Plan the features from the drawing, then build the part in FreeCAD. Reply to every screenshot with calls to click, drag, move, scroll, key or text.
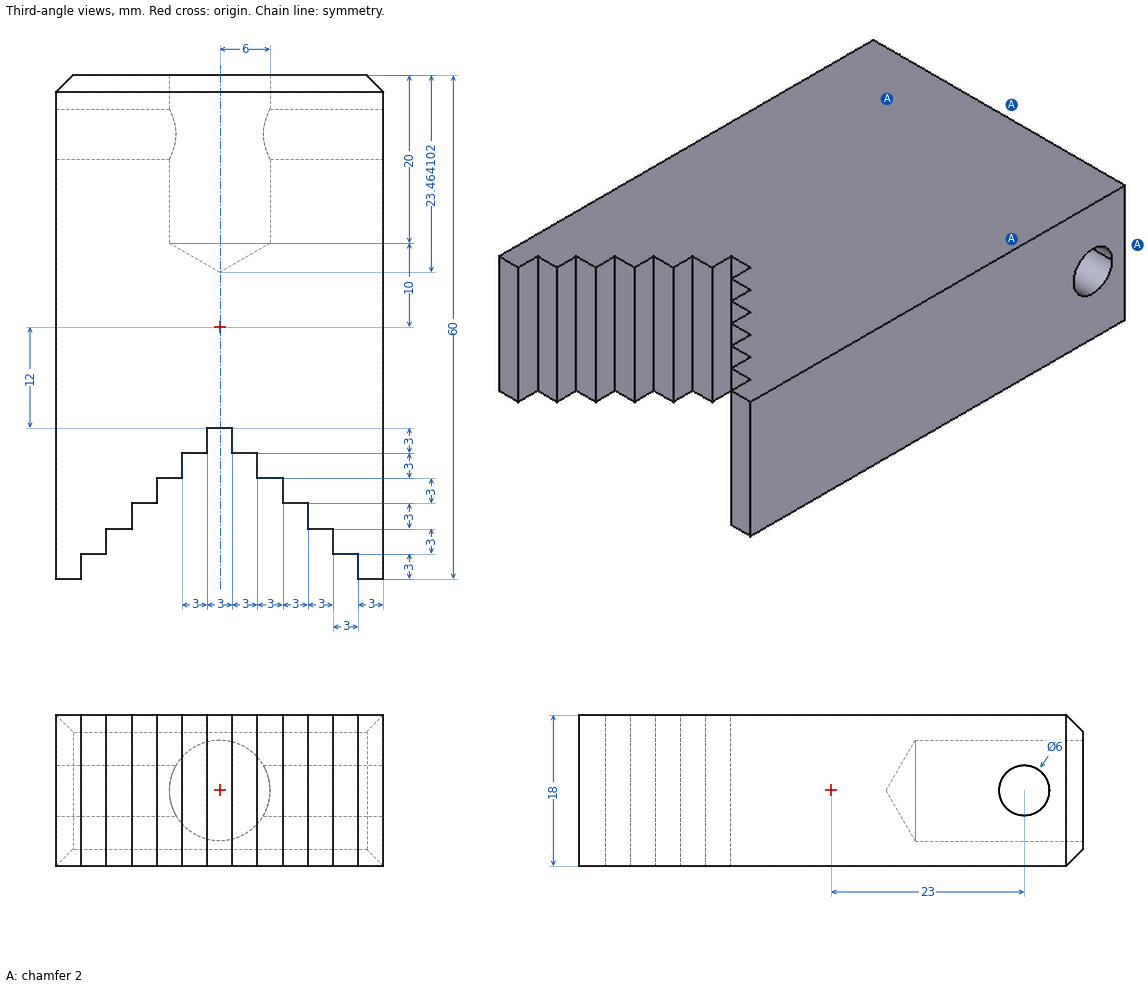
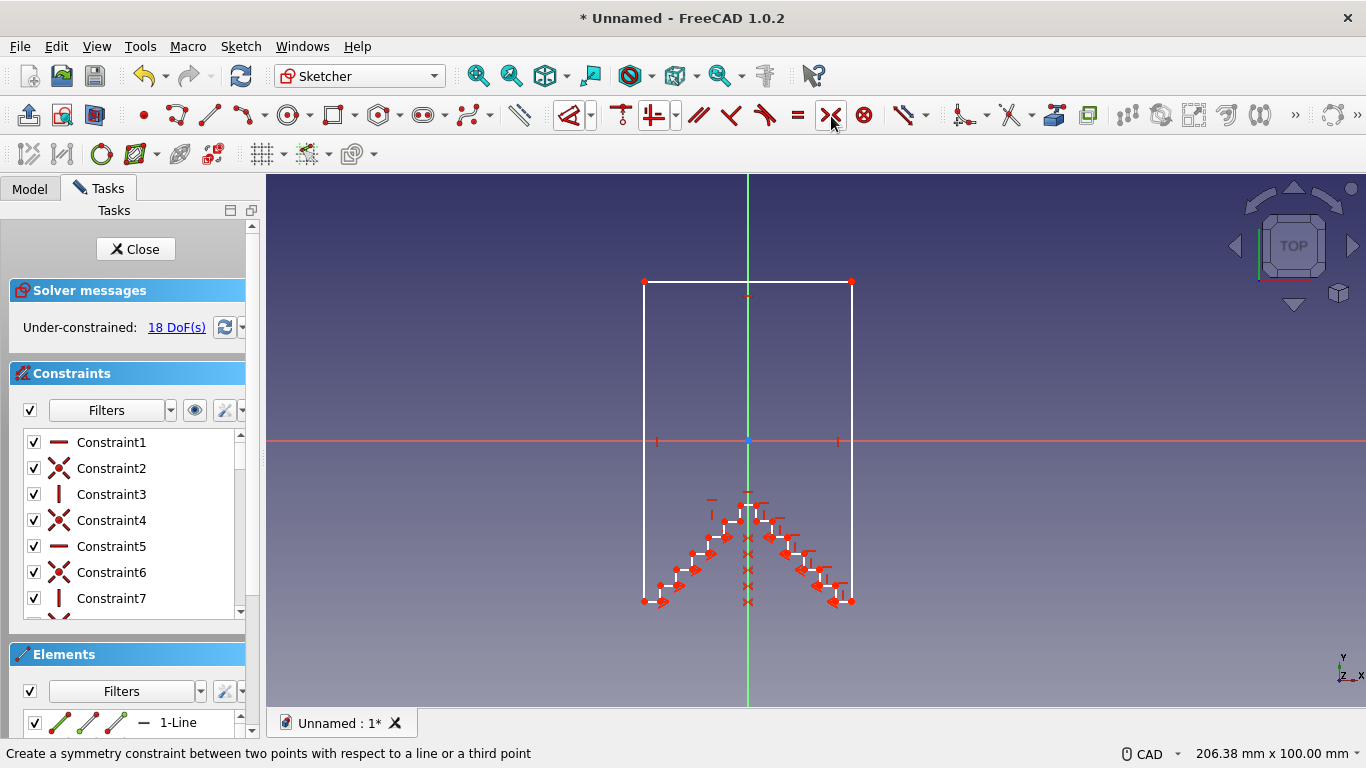
click(772, 521)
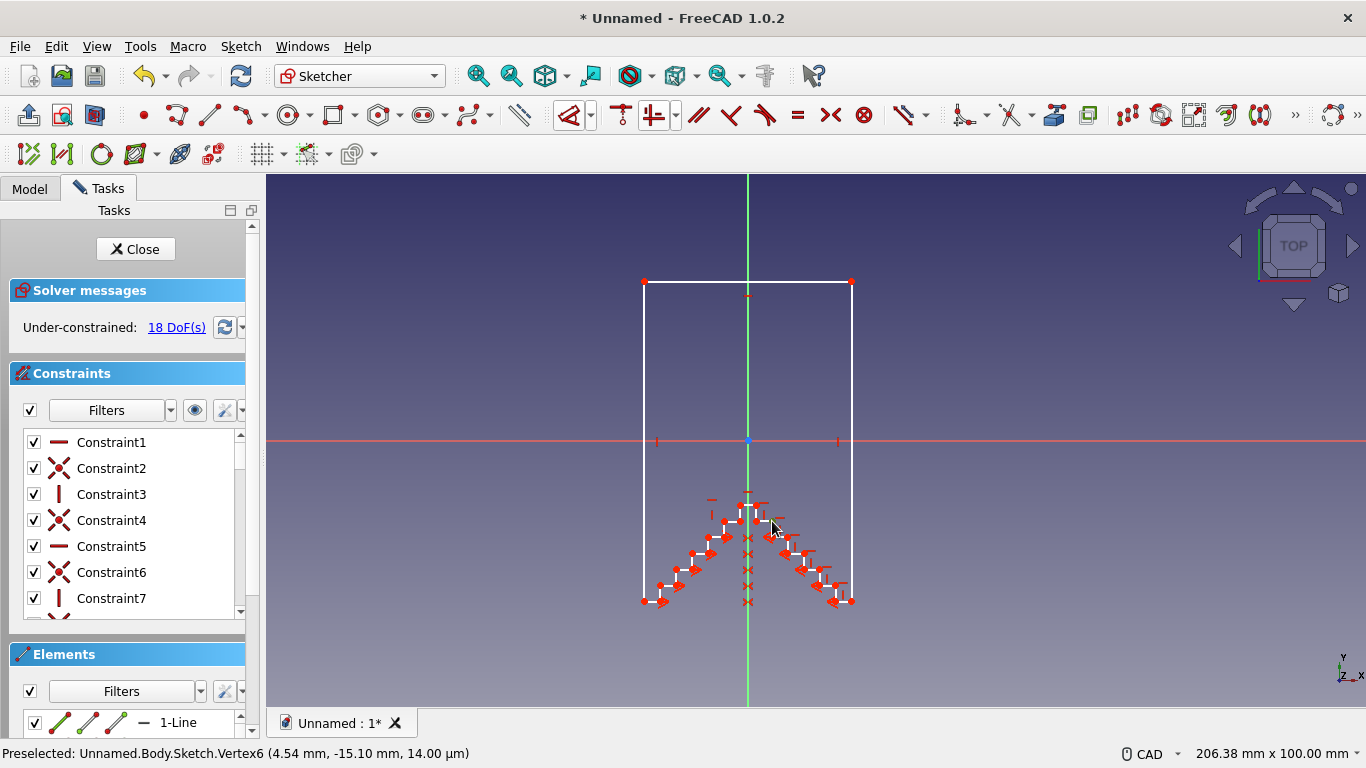
click(724, 522)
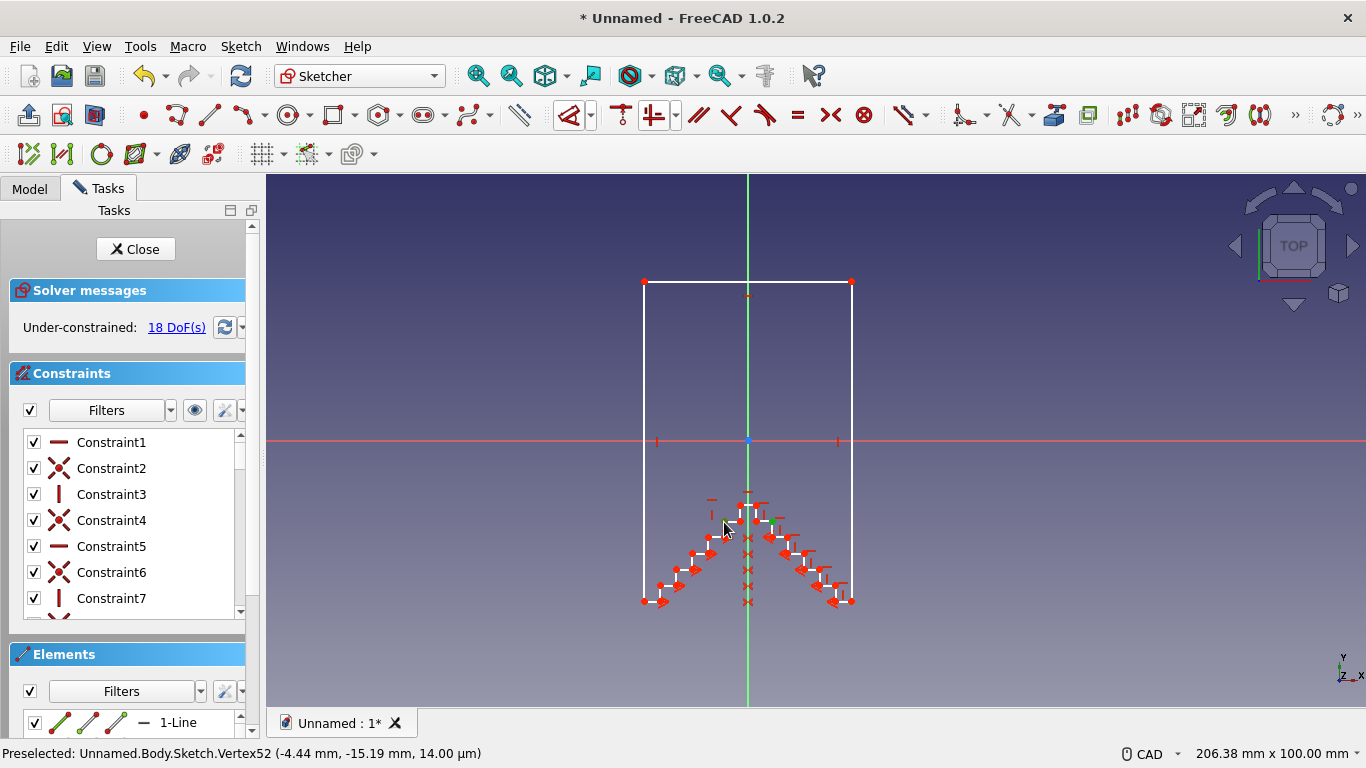
click(748, 645)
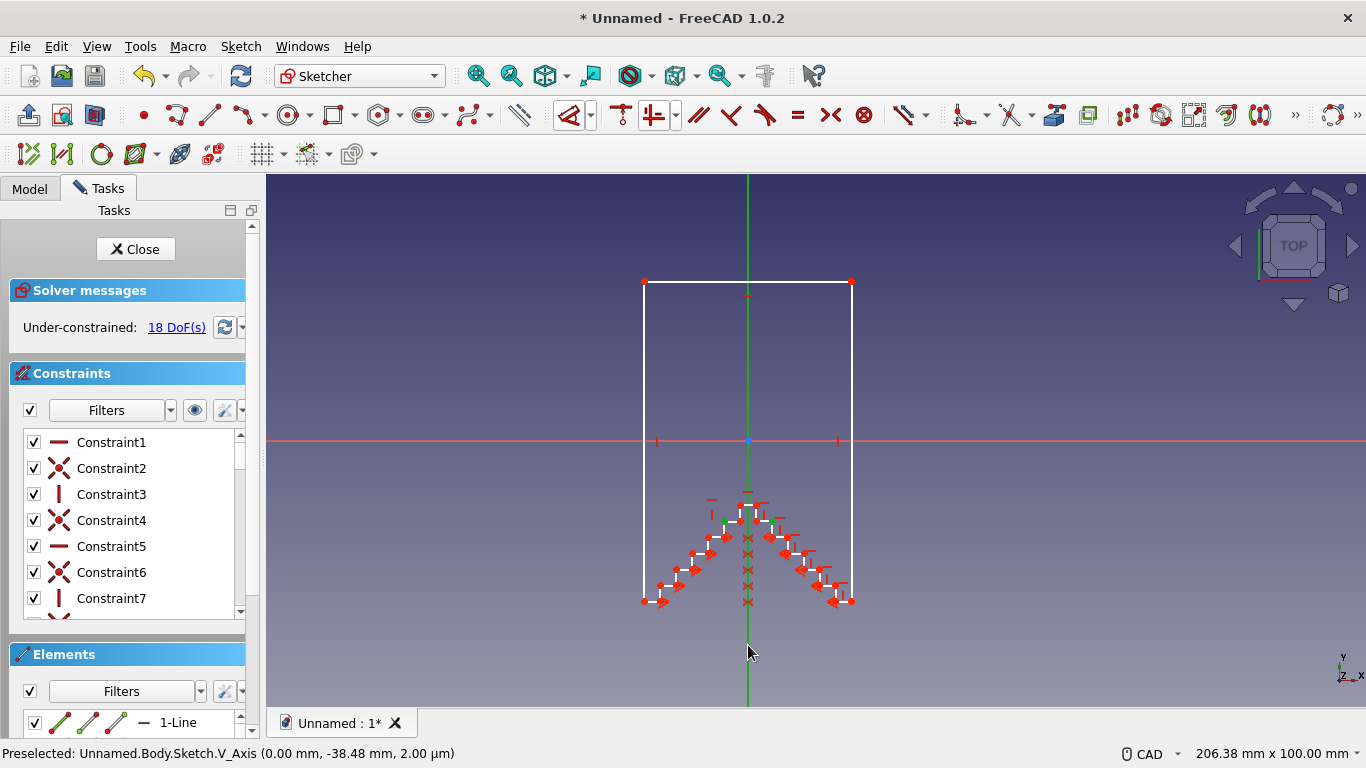
click(831, 116)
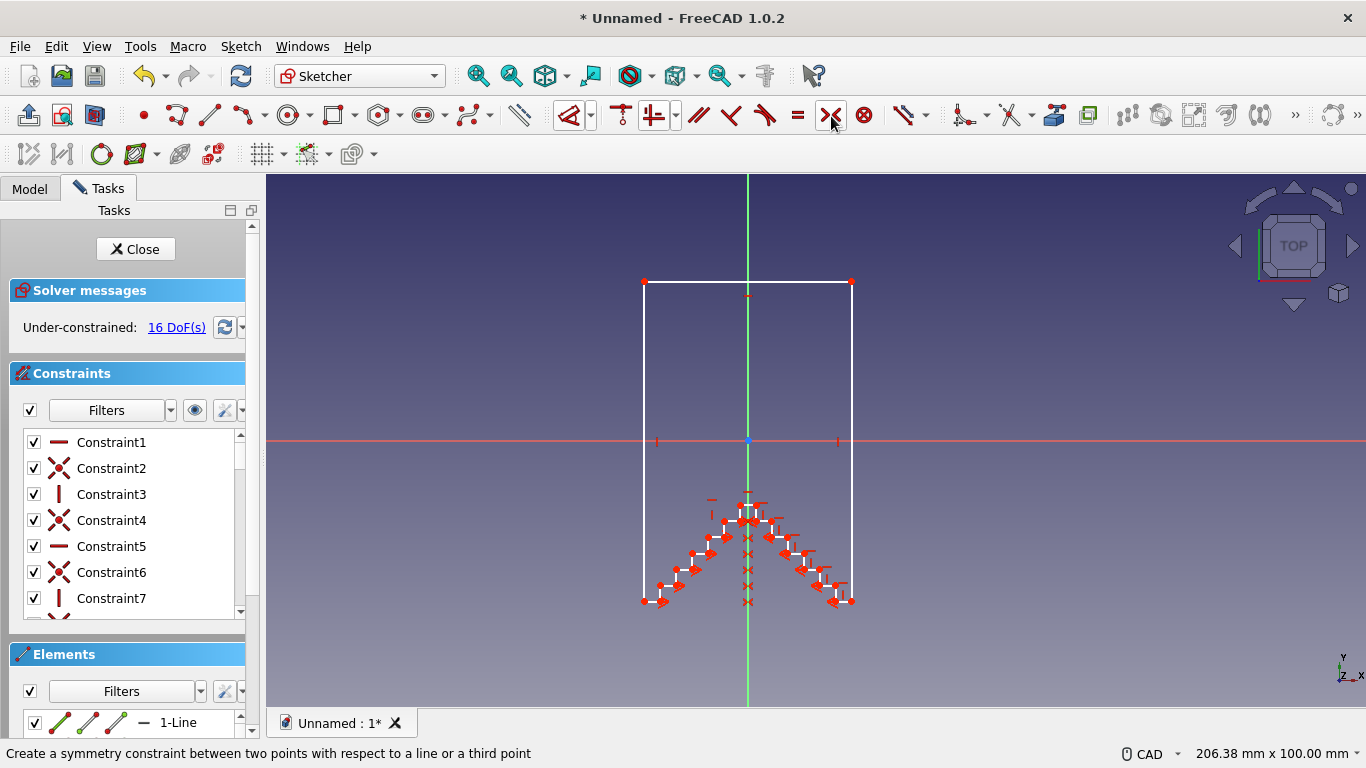
click(568, 116)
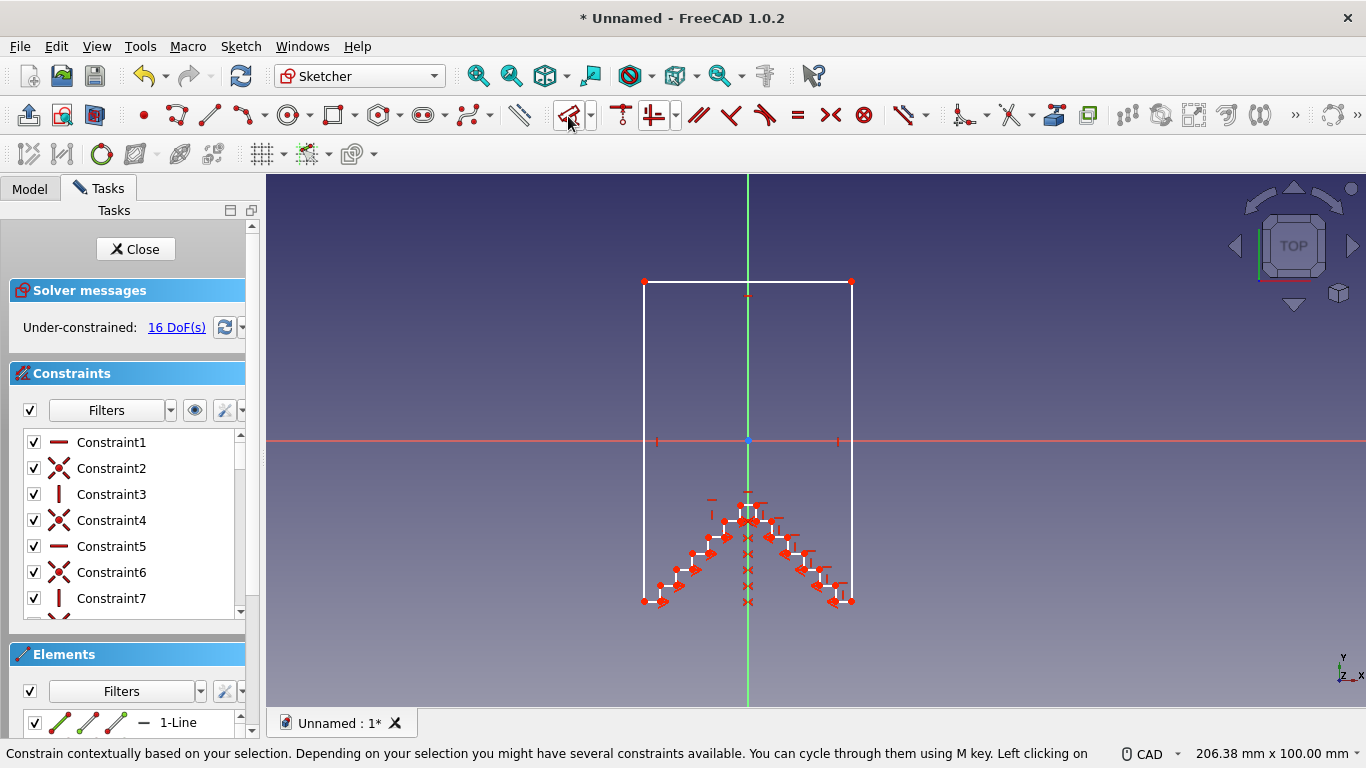
scroll(748, 505, up, 5)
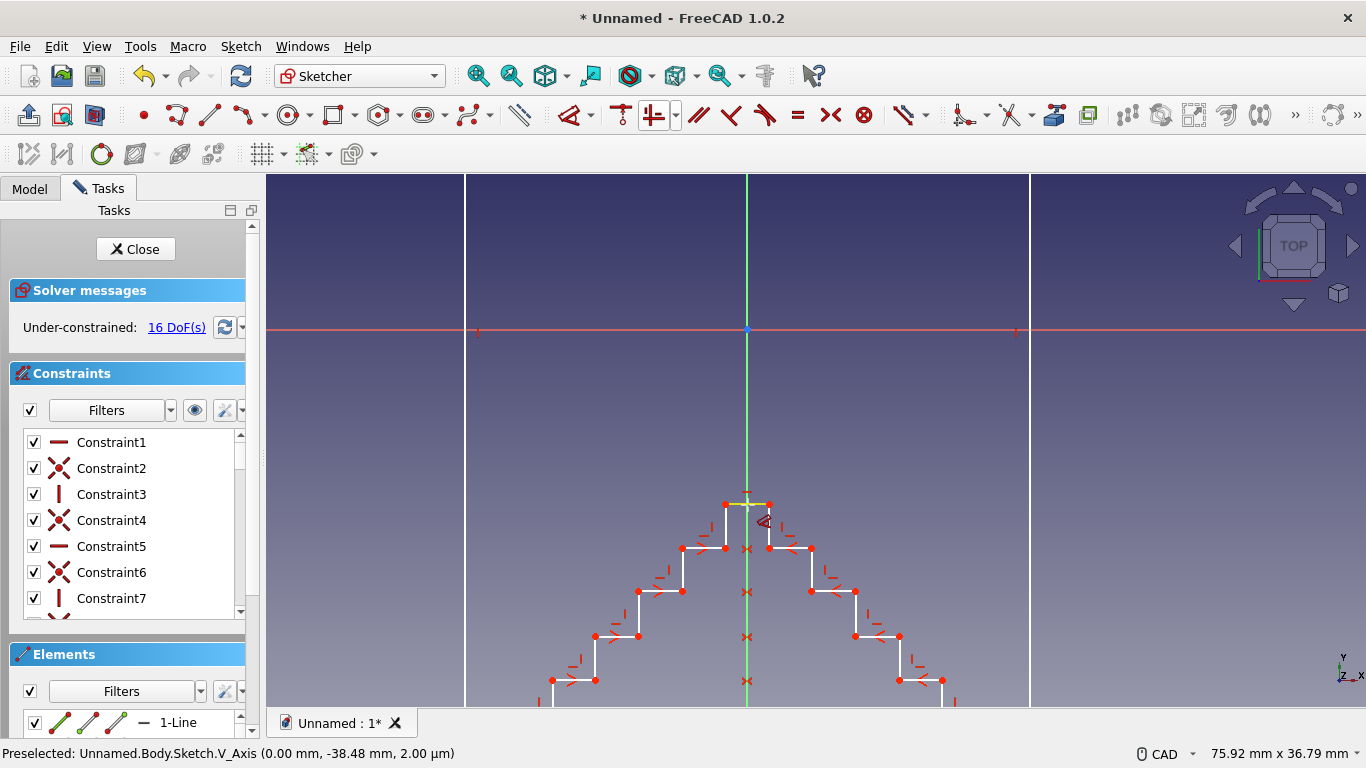
click(747, 504)
click(732, 470)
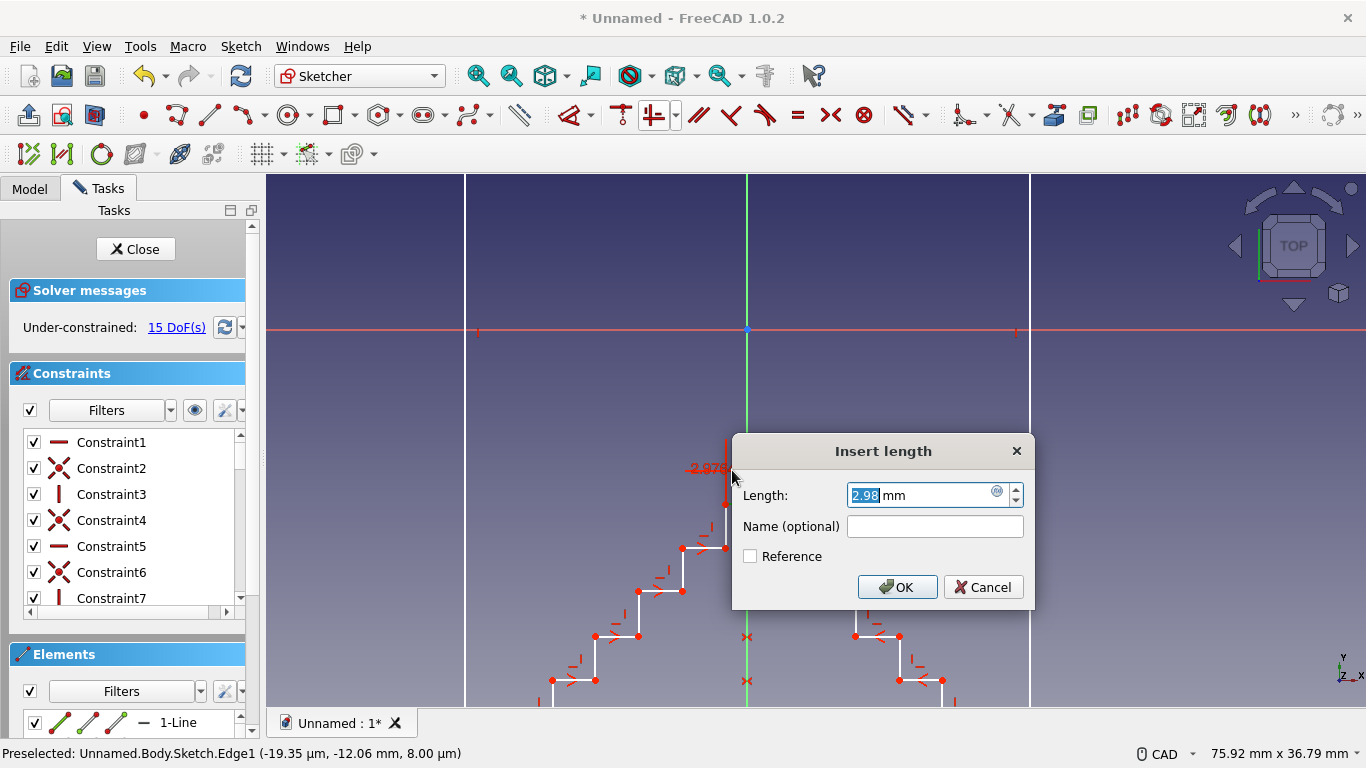
text(3)
key(Return)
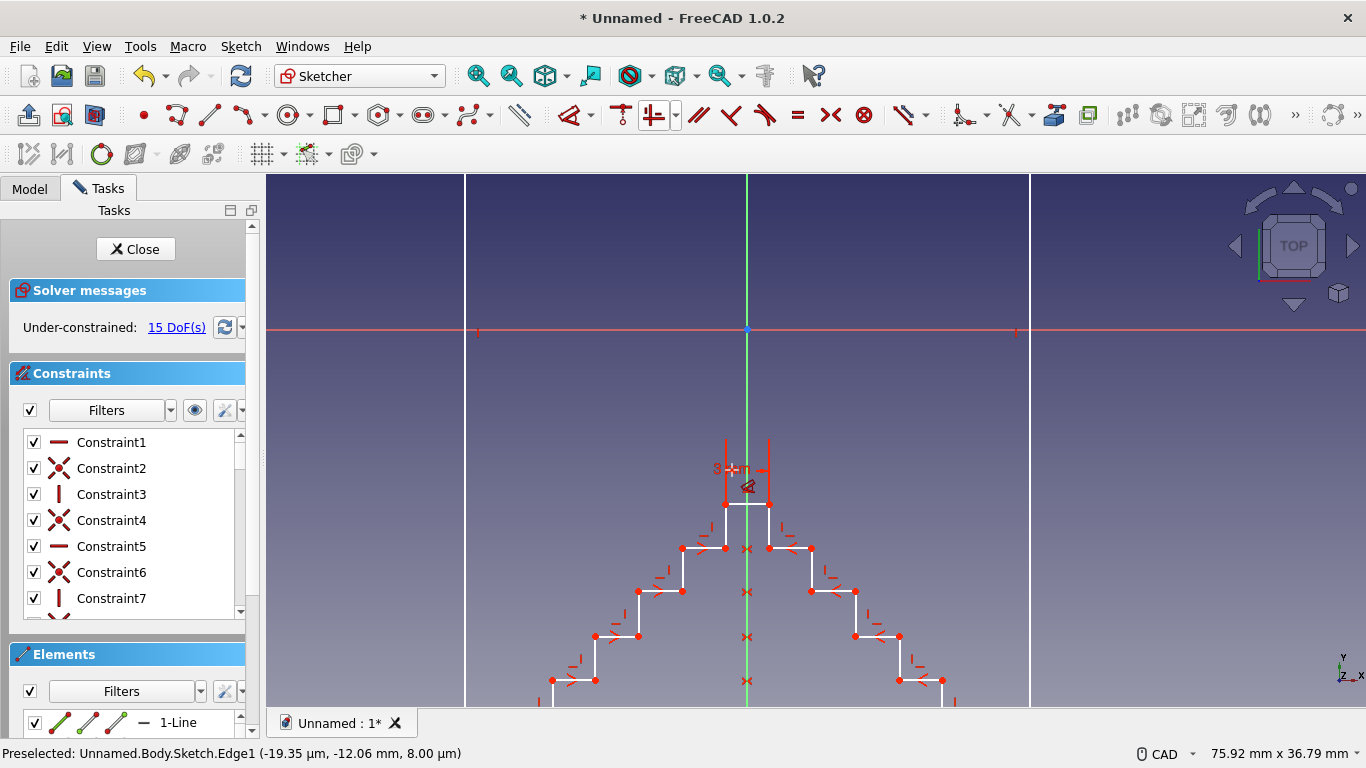
click(769, 518)
click(803, 526)